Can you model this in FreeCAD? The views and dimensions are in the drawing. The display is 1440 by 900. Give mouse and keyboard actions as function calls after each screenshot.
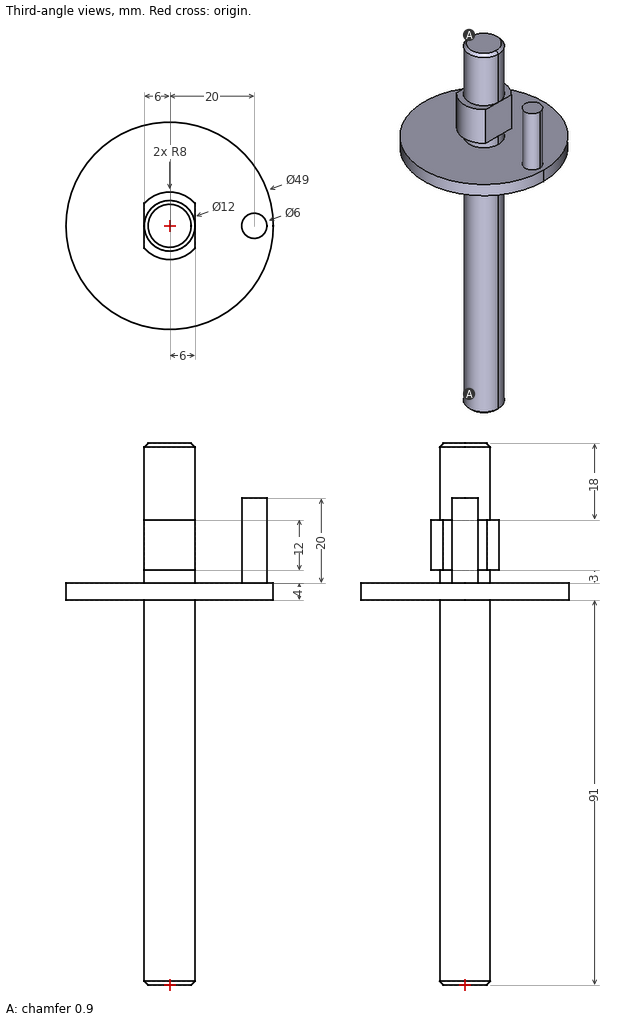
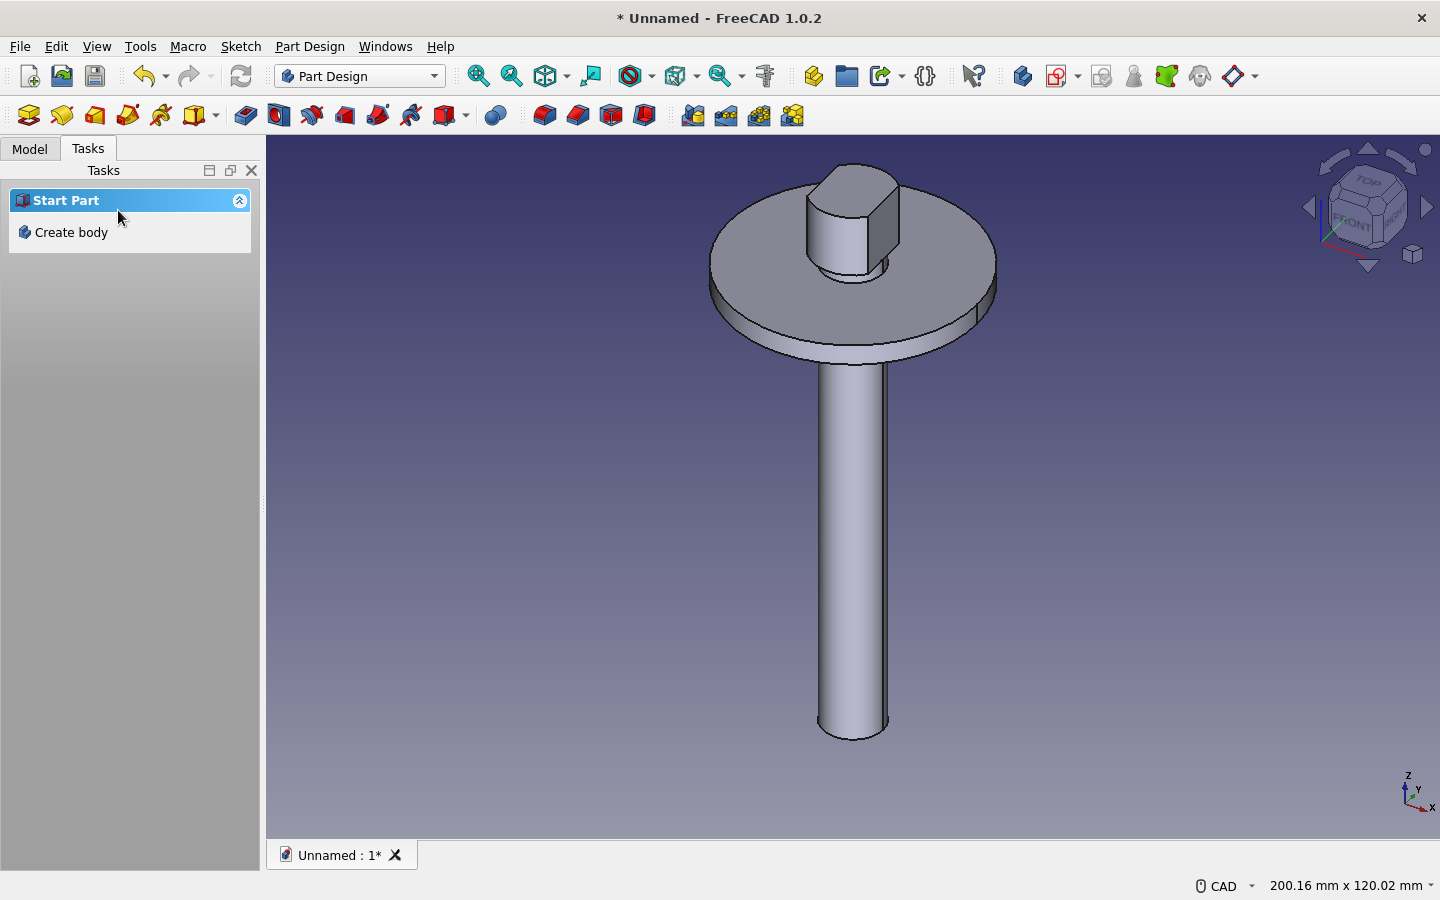
key(v)
key(f)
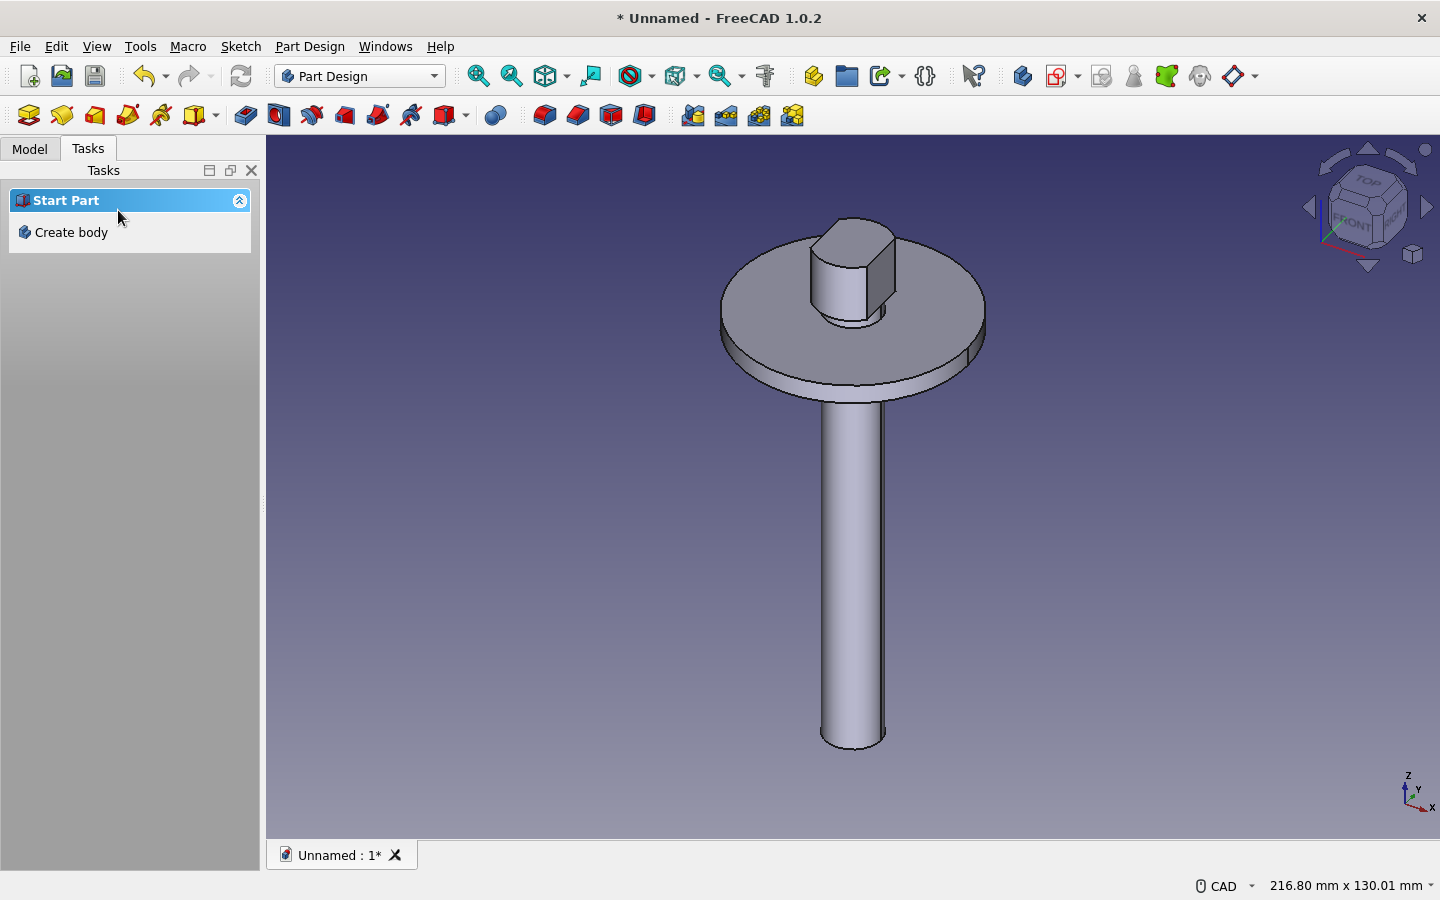
click(853, 242)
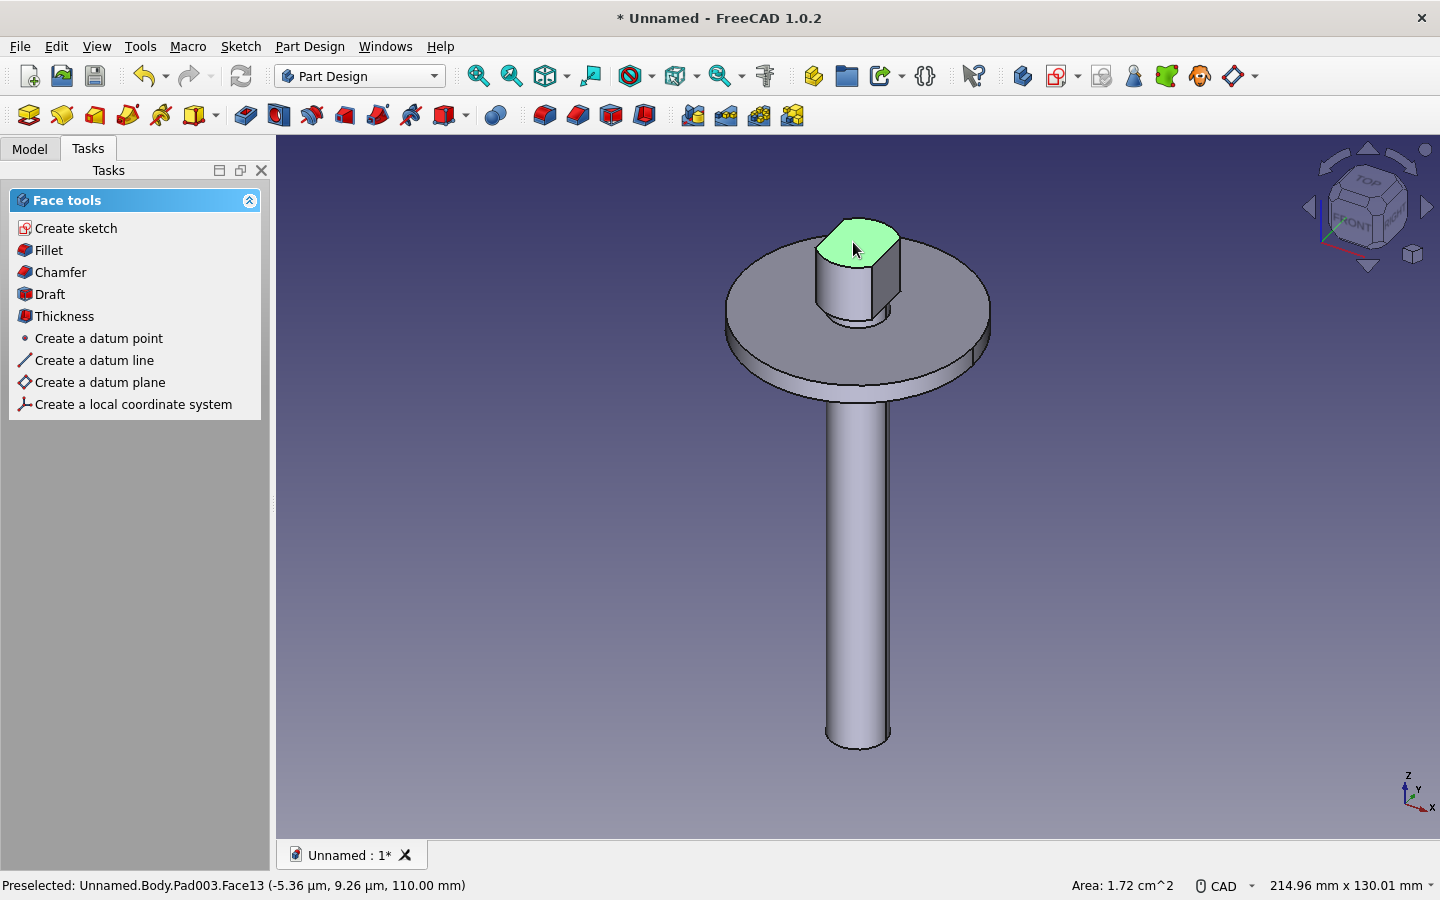
click(1056, 76)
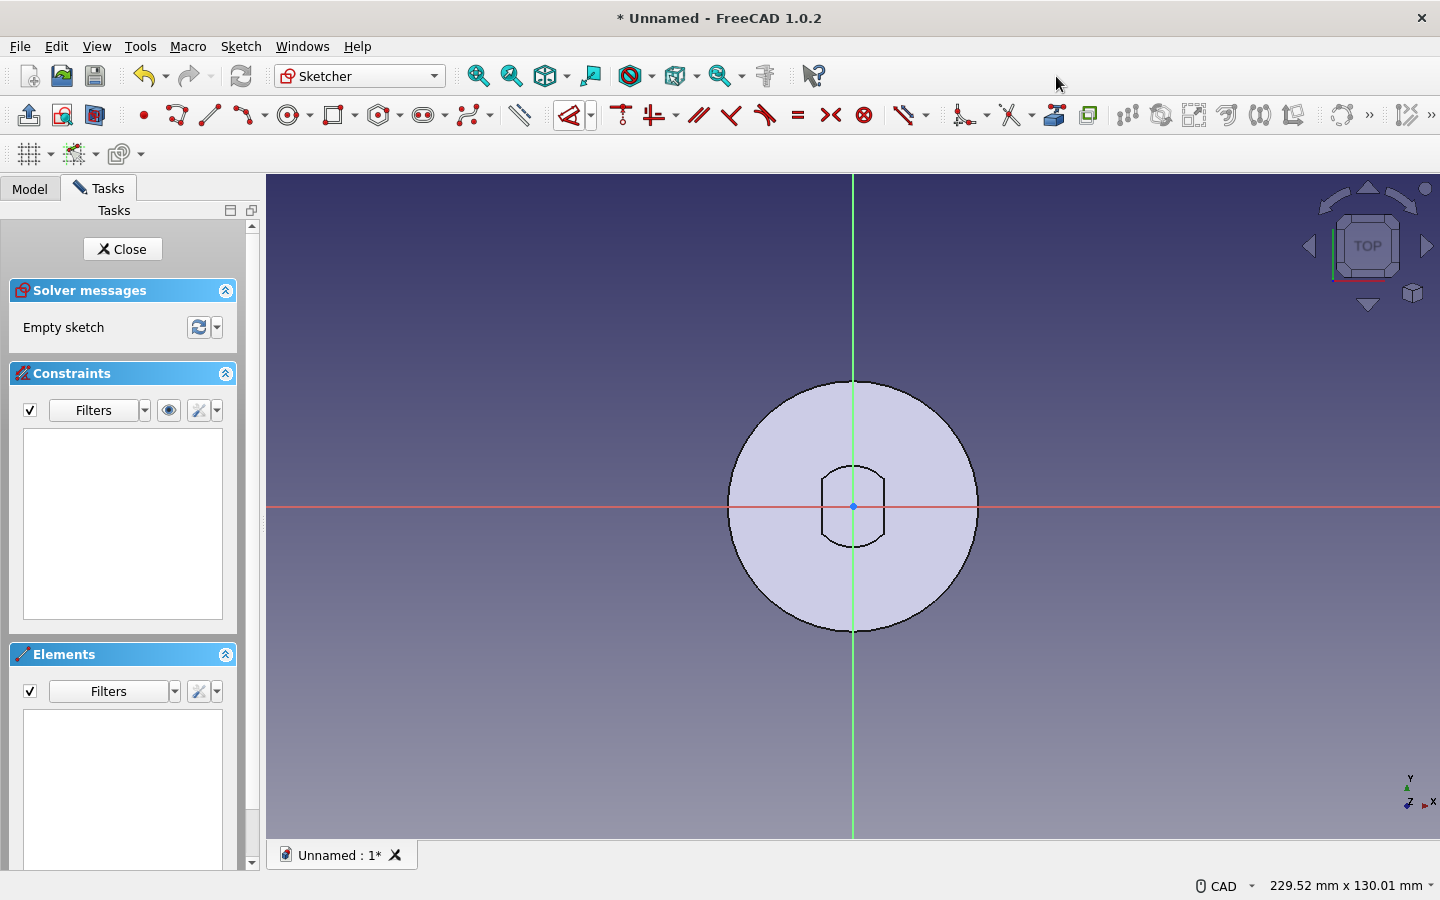
scroll(864, 506, up, 10)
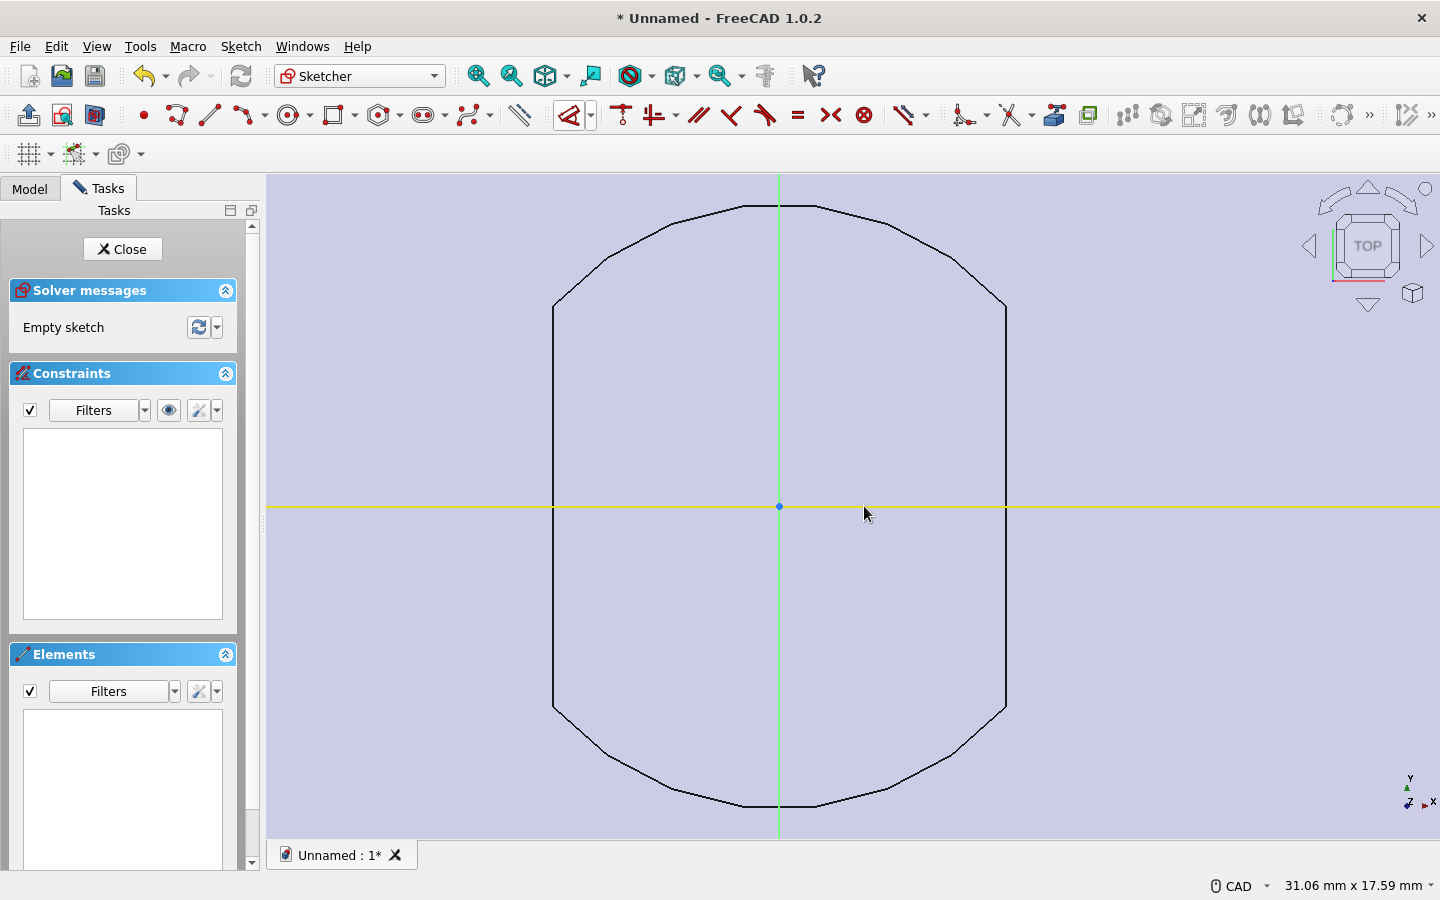
click(288, 116)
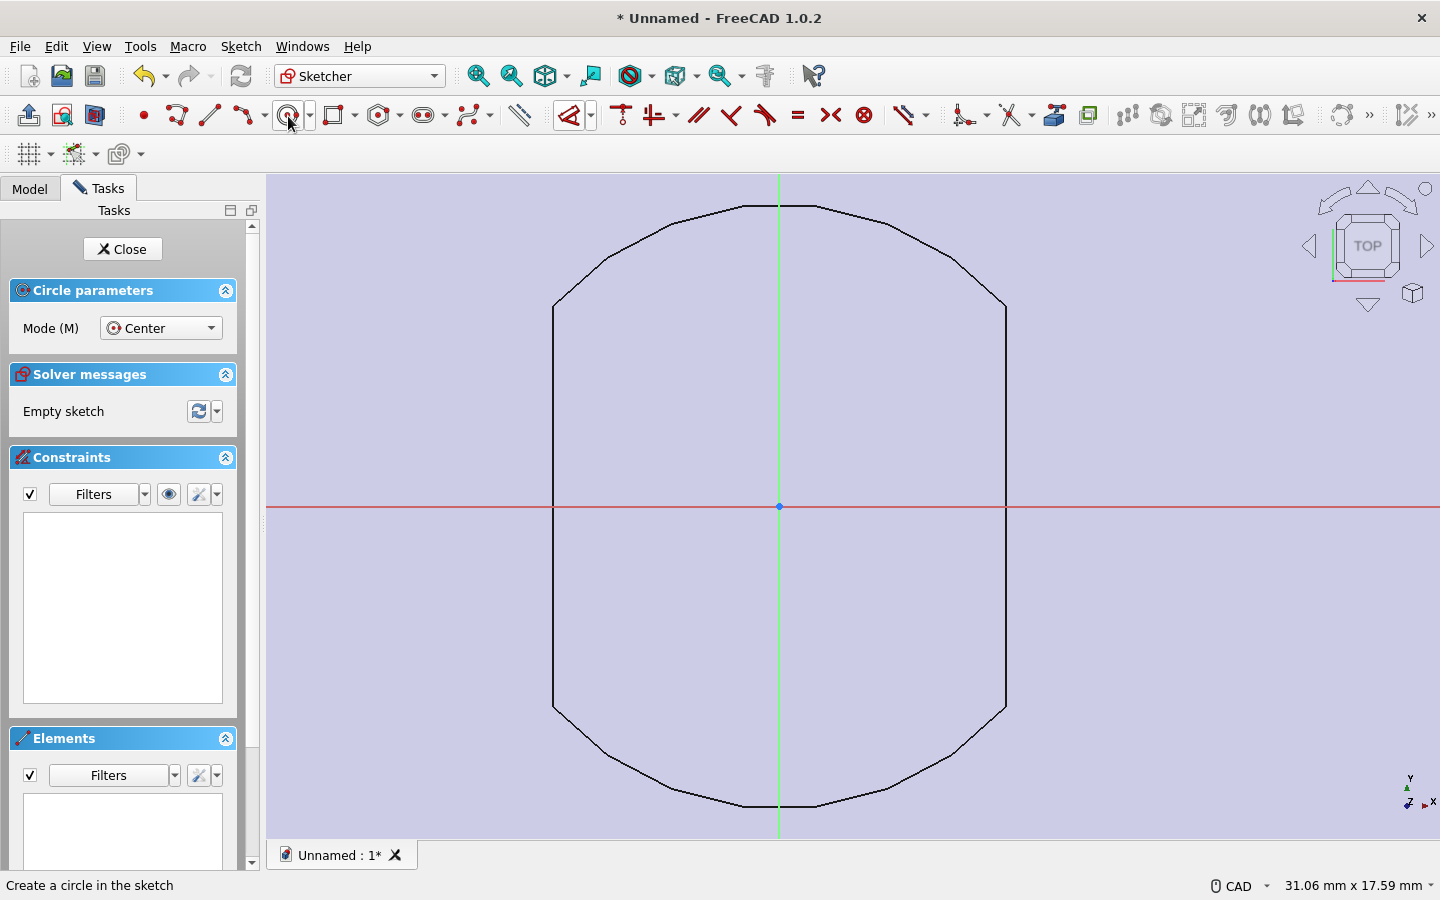
click(779, 506)
click(940, 346)
key(Escape)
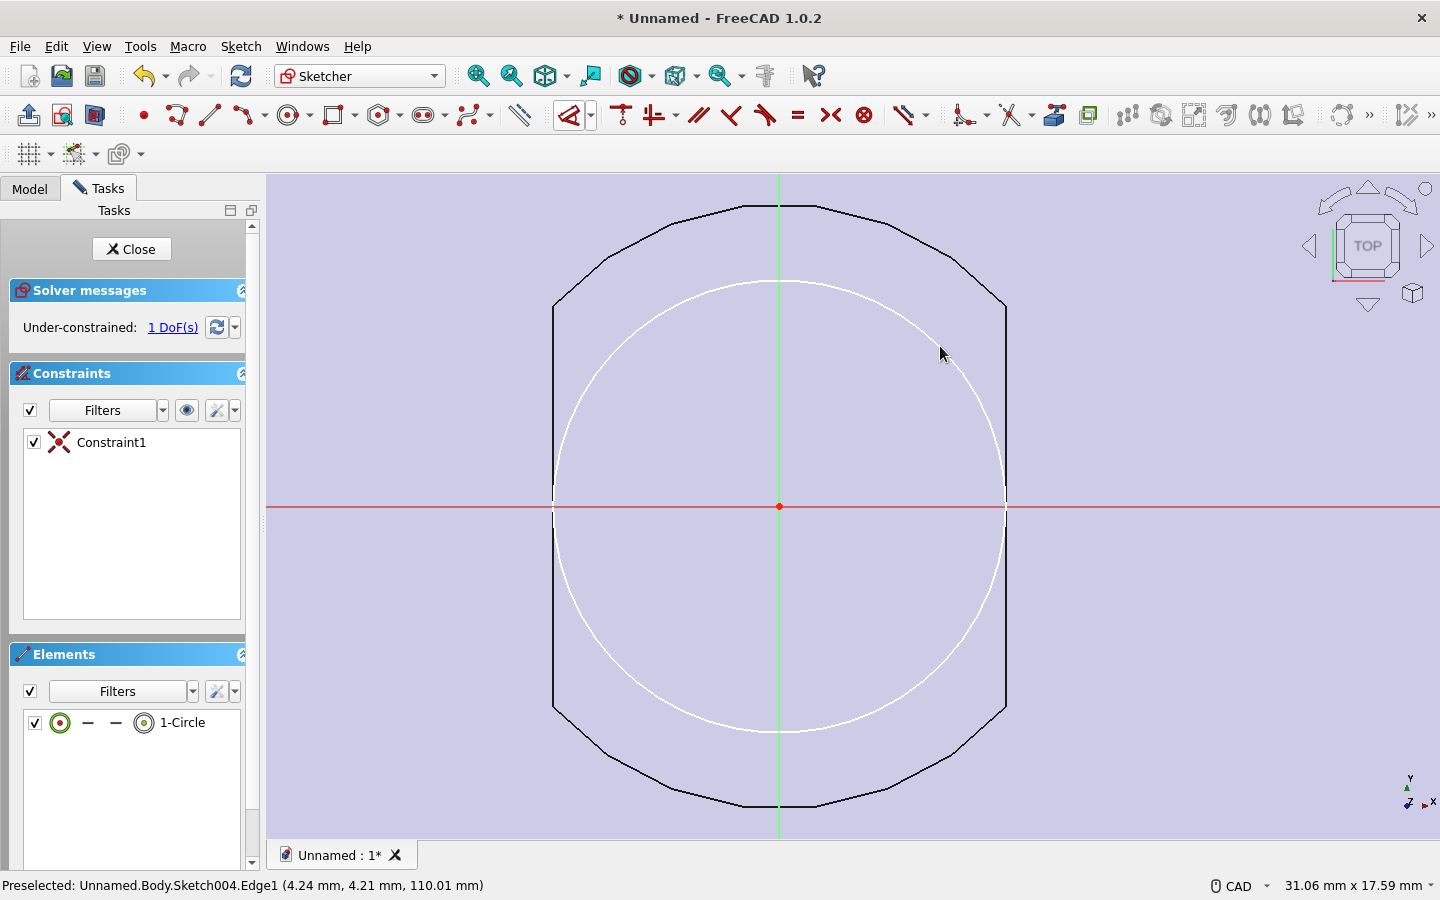
click(939, 346)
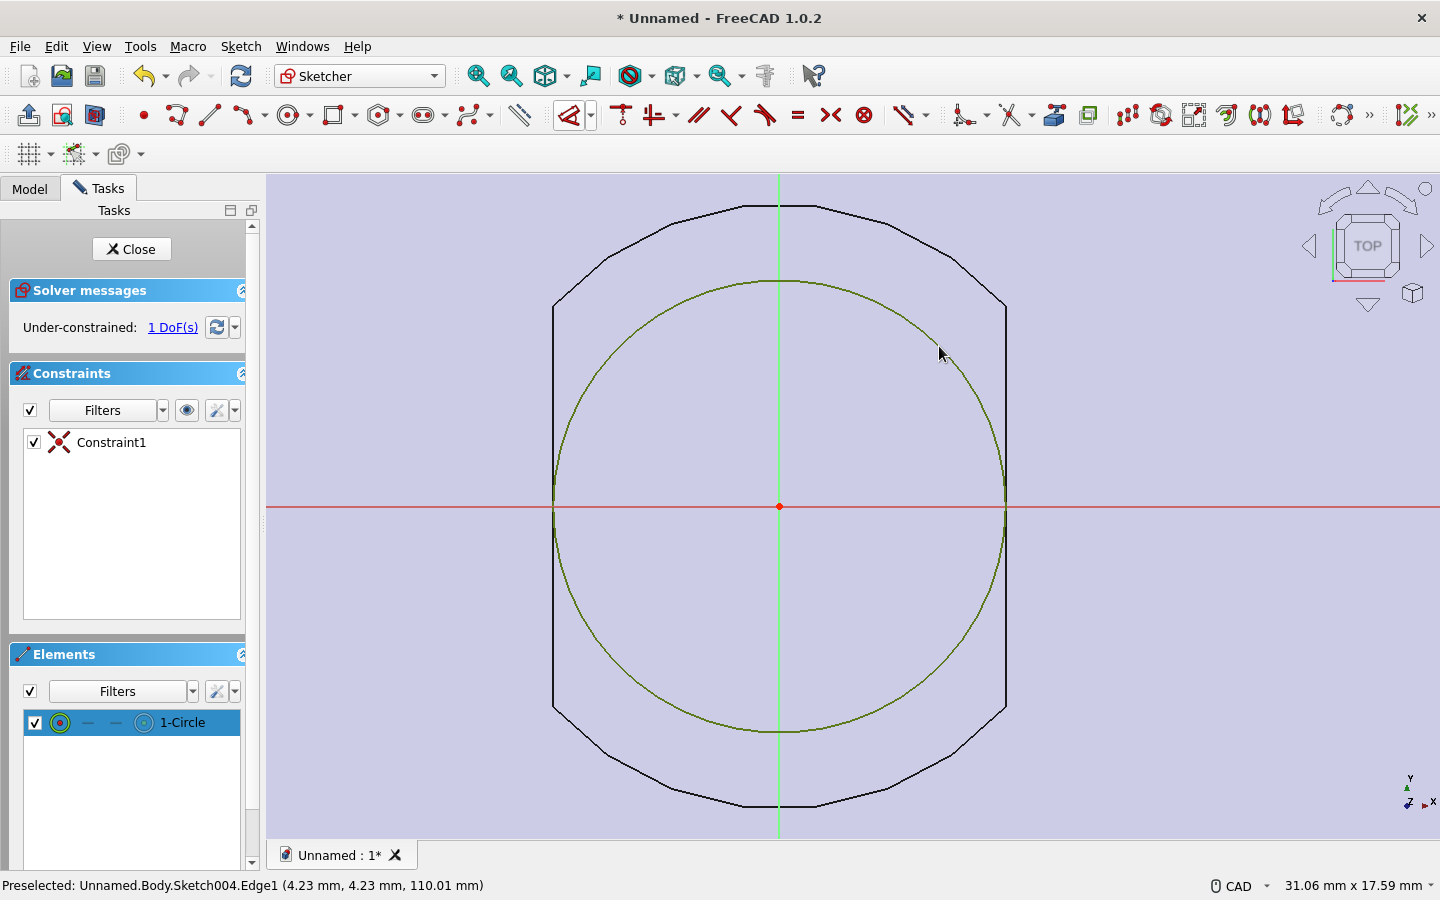
key(k)
key(o)